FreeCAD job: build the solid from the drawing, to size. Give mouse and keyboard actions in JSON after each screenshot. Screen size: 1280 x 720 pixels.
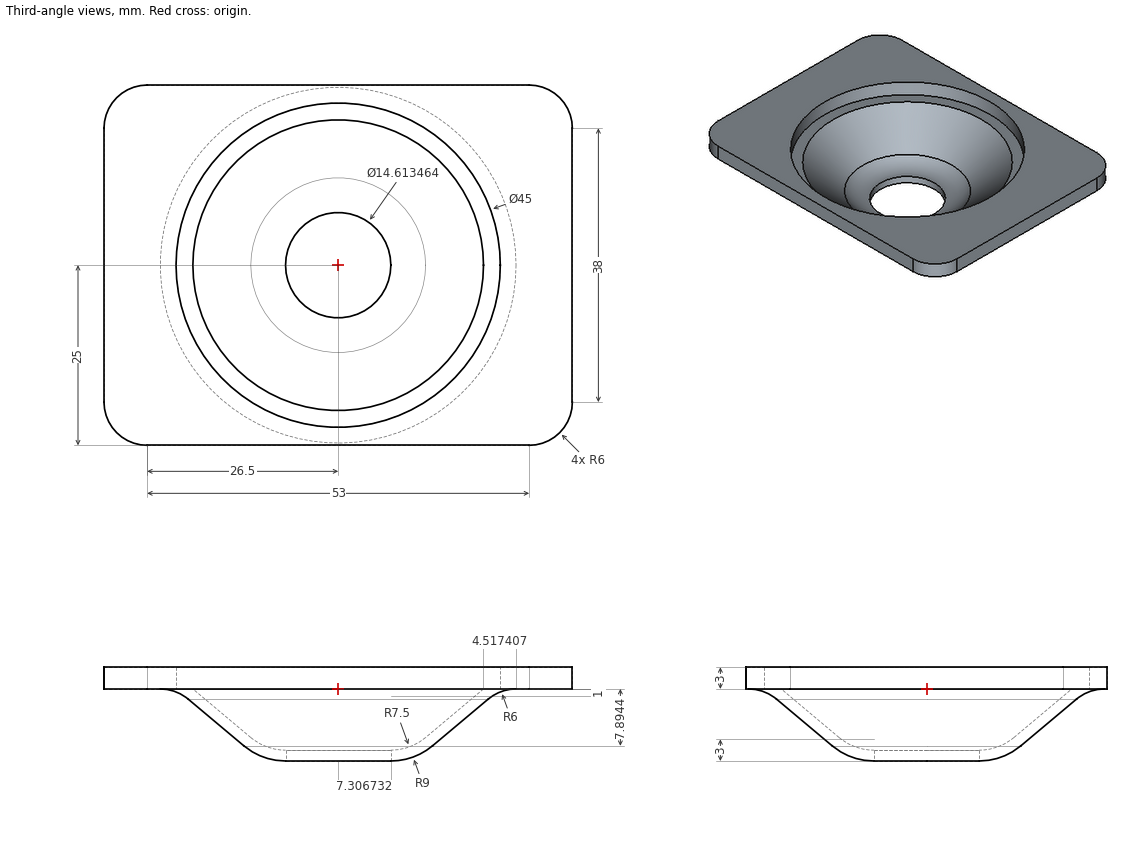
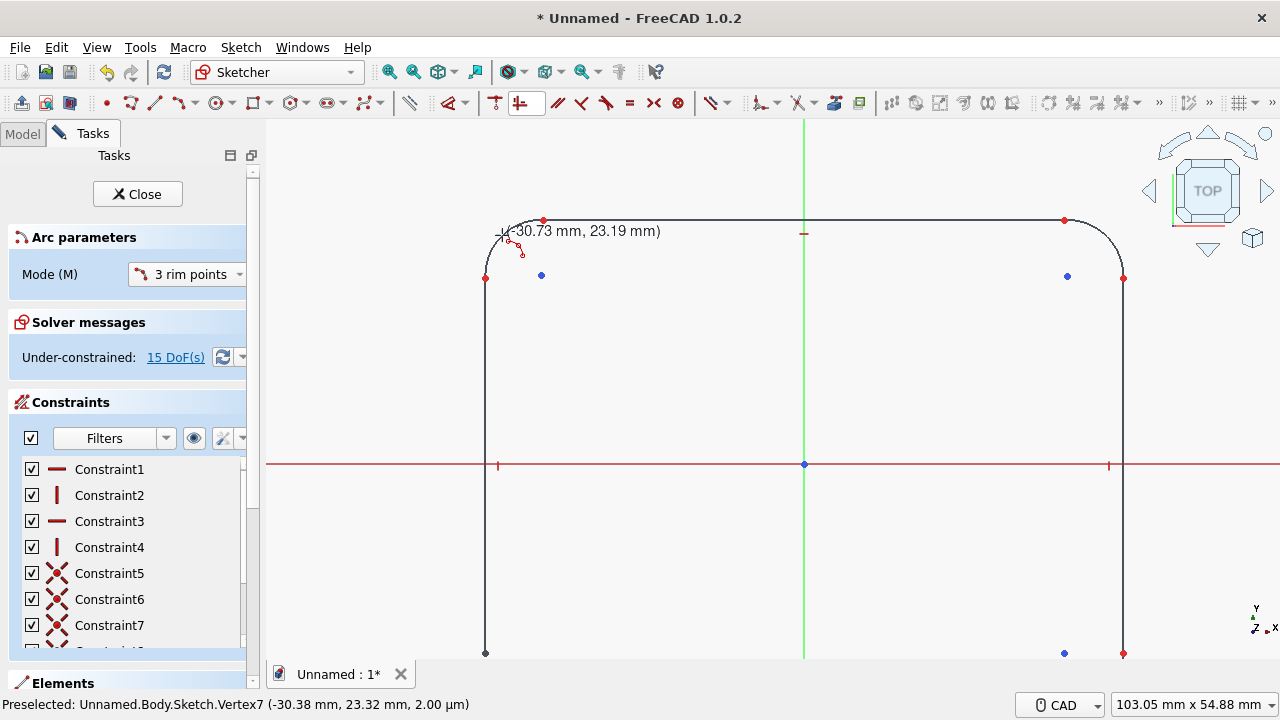
{"action": "scroll", "coordinate": [501, 236], "scroll_direction": "down", "scroll_amount": 2}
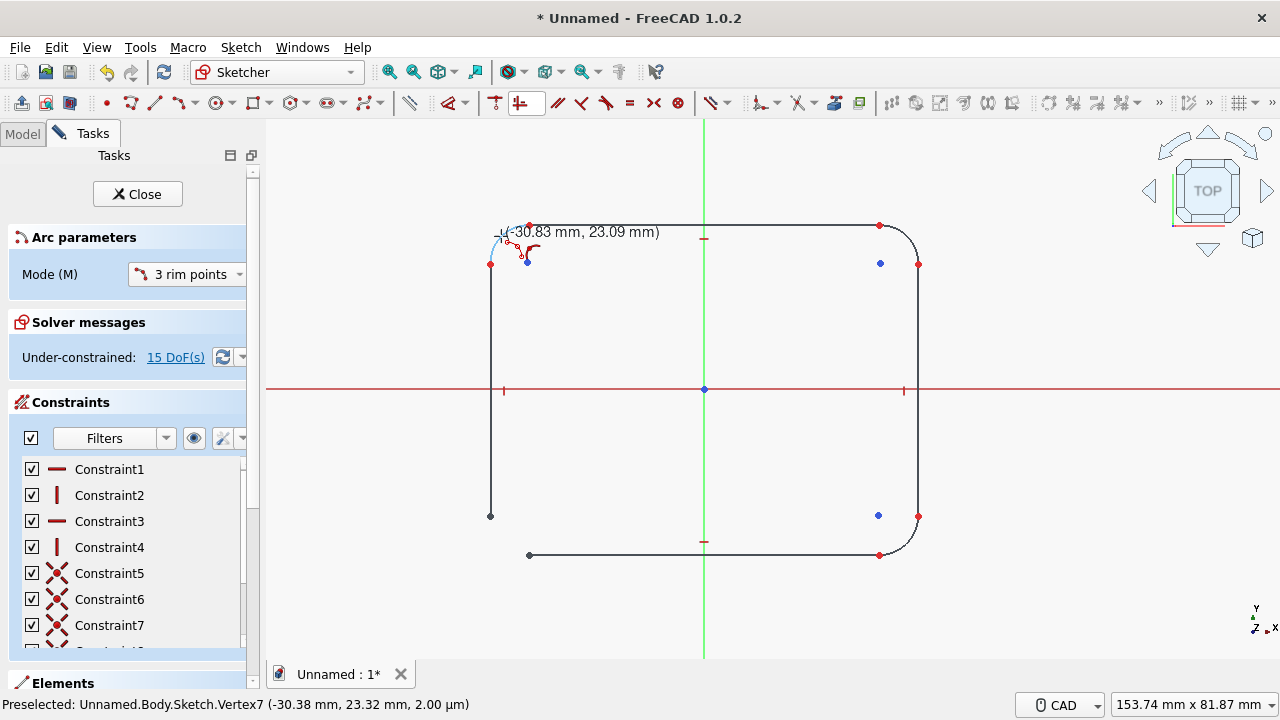
{"action": "left_click", "coordinate": [491, 516]}
{"action": "left_click", "coordinate": [530, 555]}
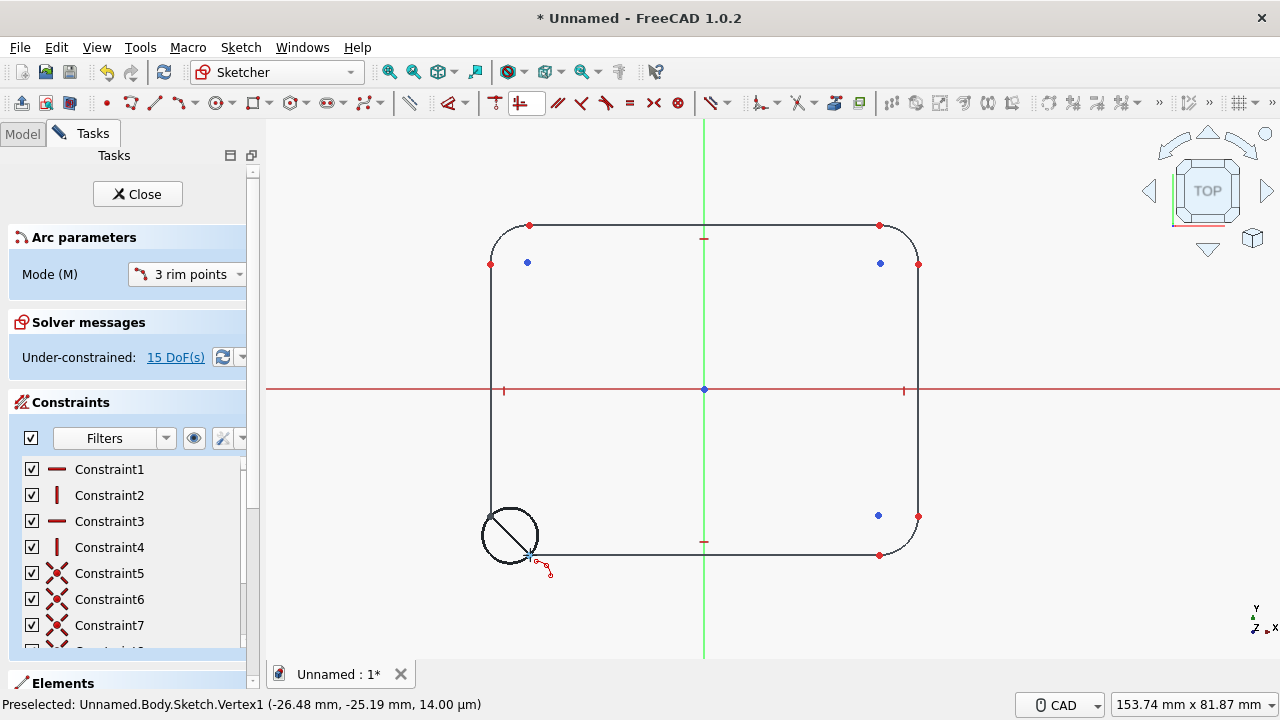
{"action": "scroll", "coordinate": [502, 542], "scroll_direction": "up", "scroll_amount": 2}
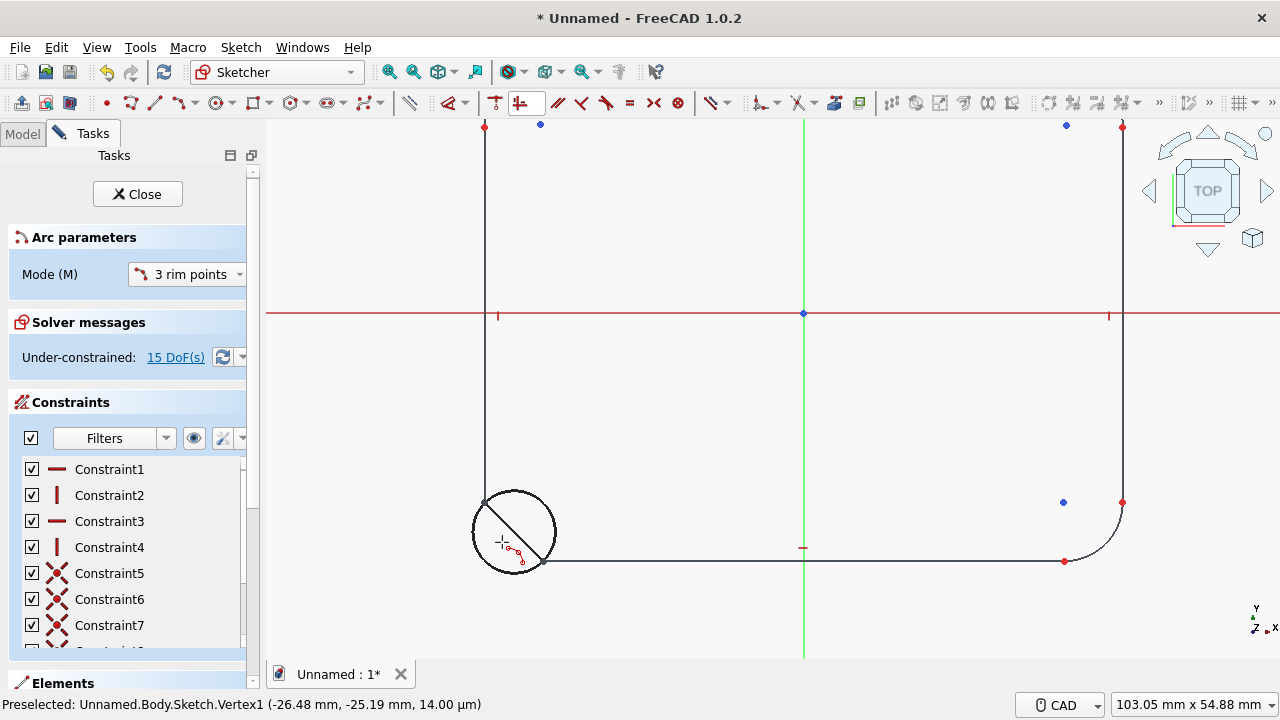
{"action": "left_click", "coordinate": [501, 542]}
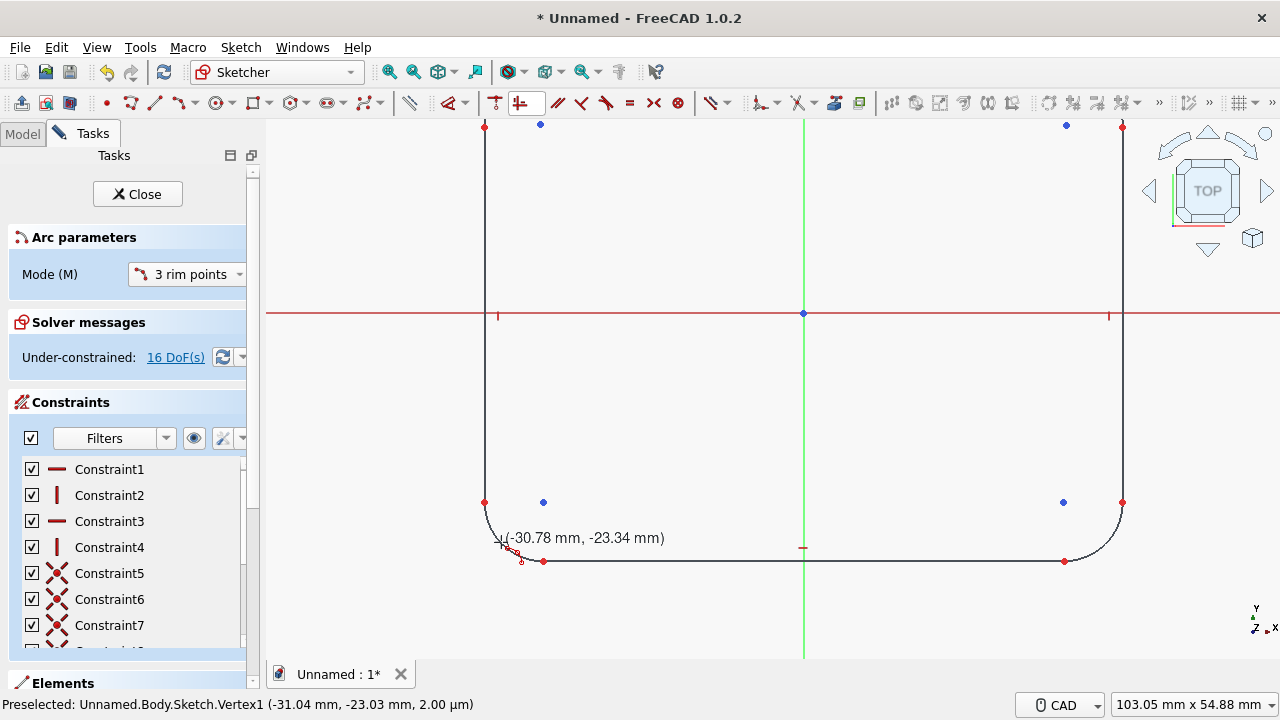
{"action": "key", "text": "g c"}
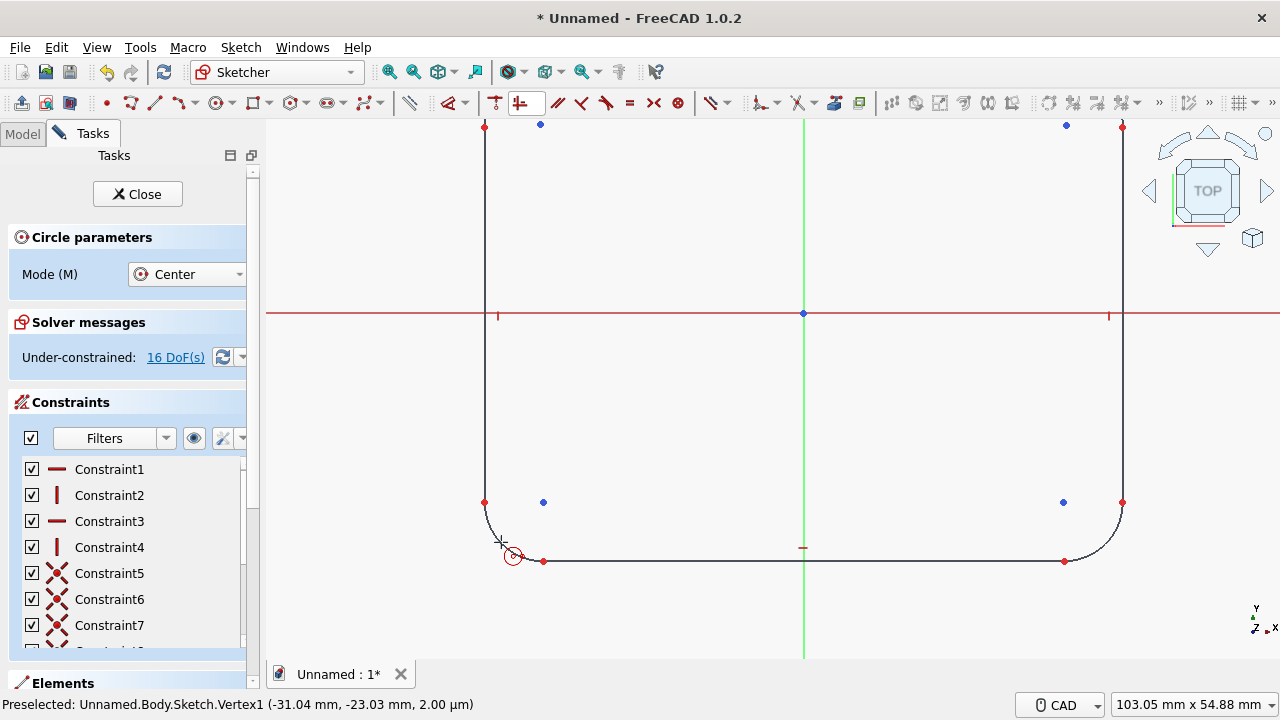
{"action": "left_click", "coordinate": [804, 313]}
{"action": "mouse_move", "coordinate": [960, 157]}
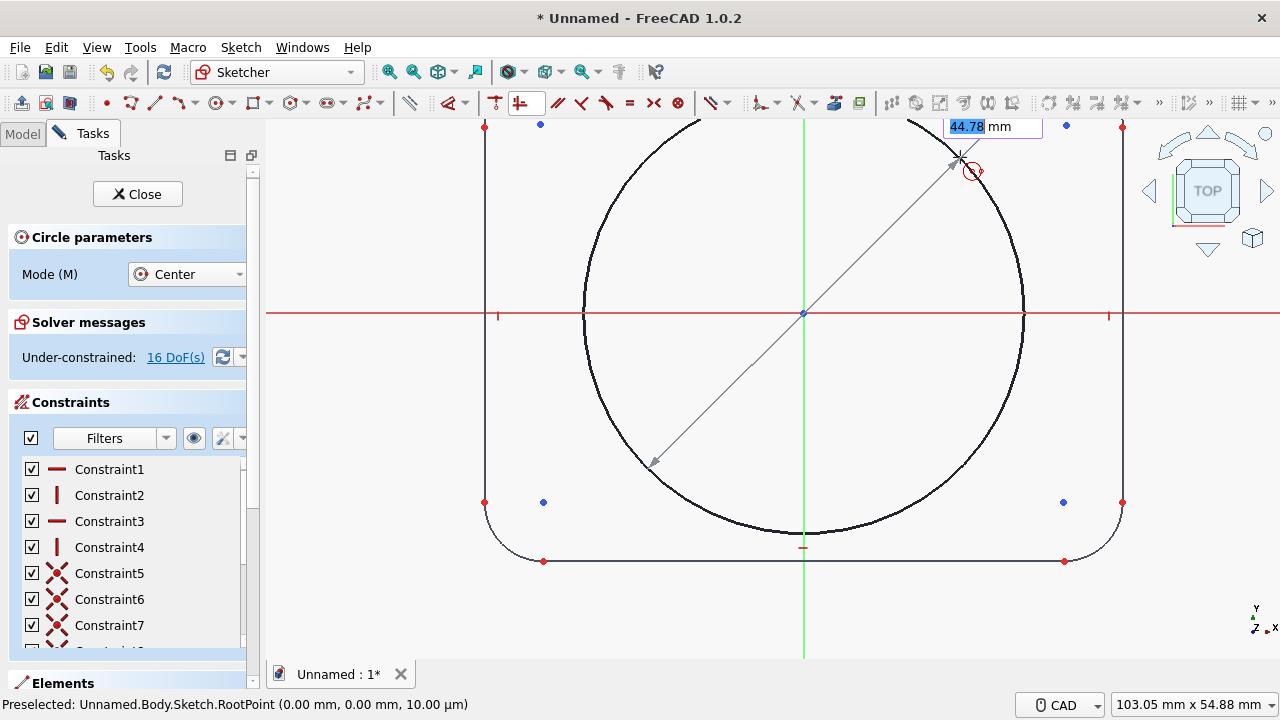
{"action": "type", "text": "45"}
{"action": "key", "text": "Return"}
{"action": "key", "text": "Escape"}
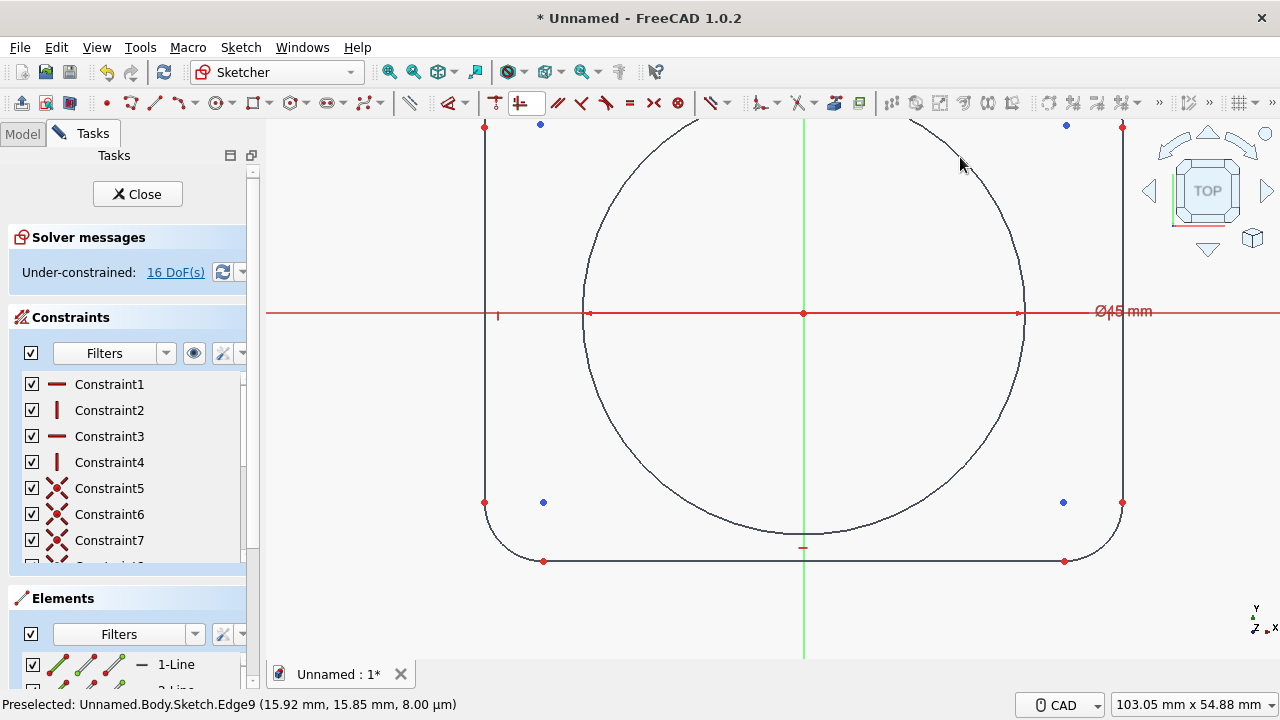
{"action": "left_click", "coordinate": [700, 561]}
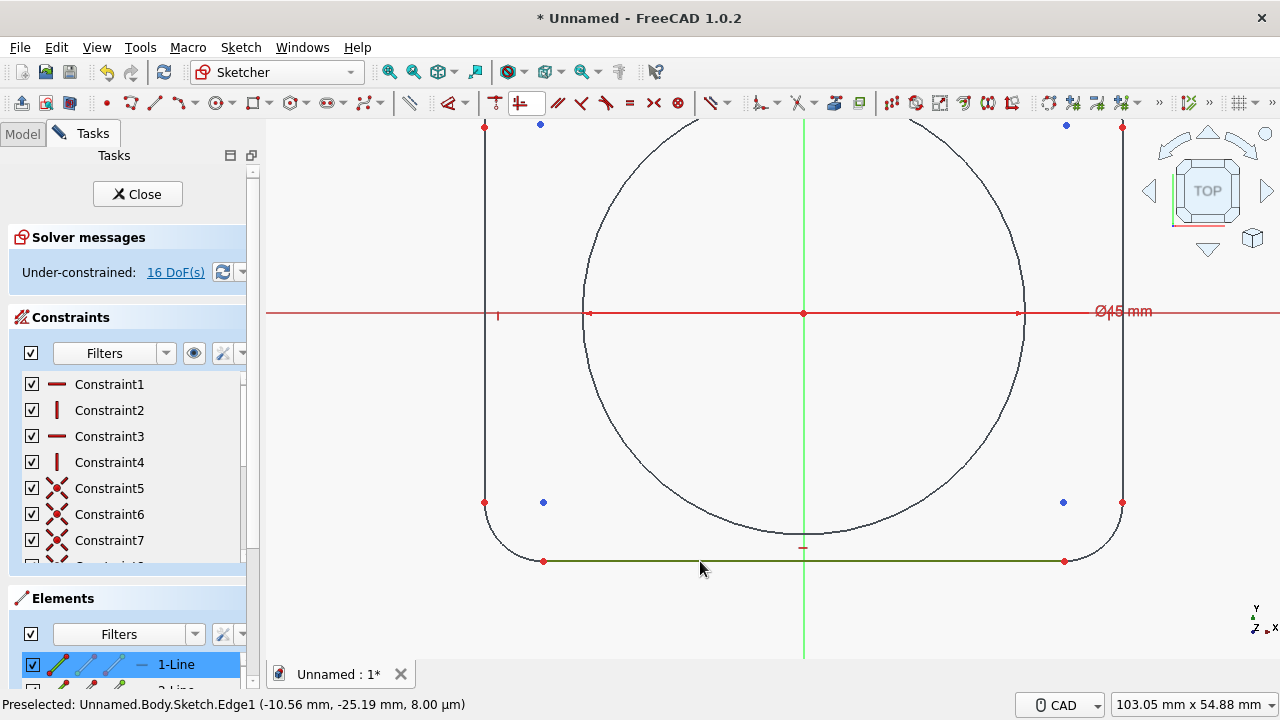
{"action": "left_click", "coordinate": [1091, 555]}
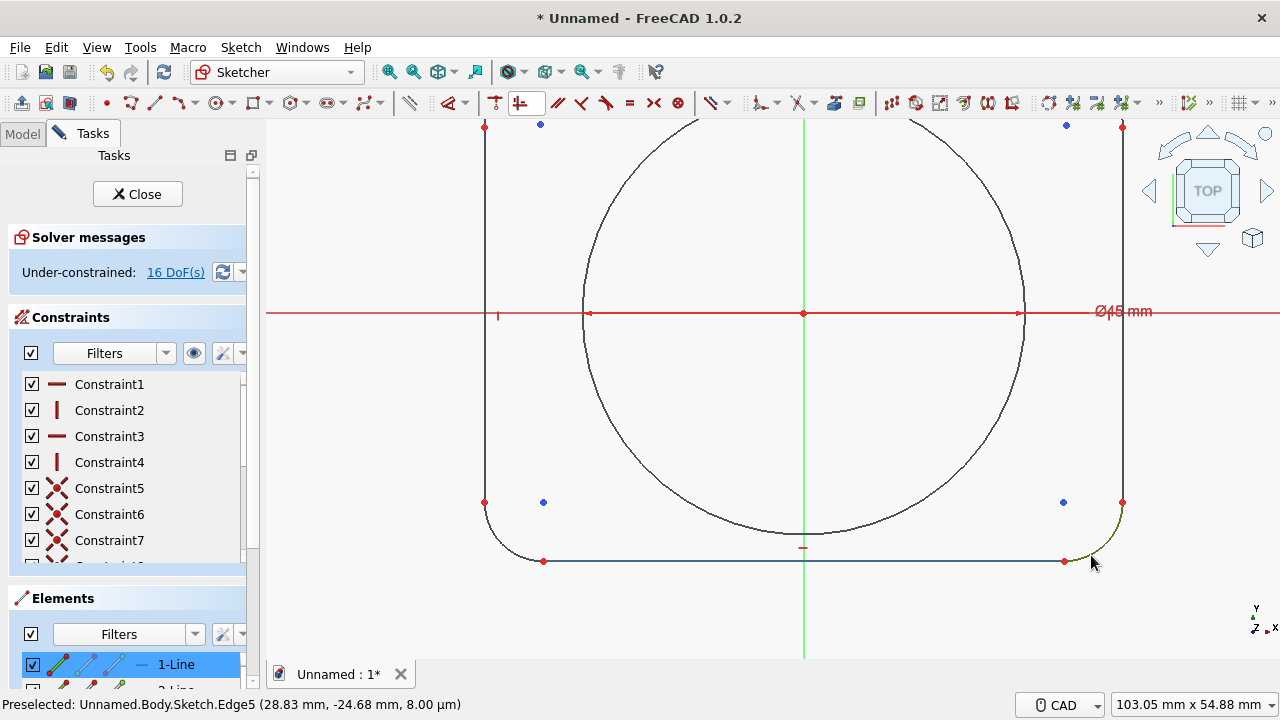
{"action": "key", "text": "t"}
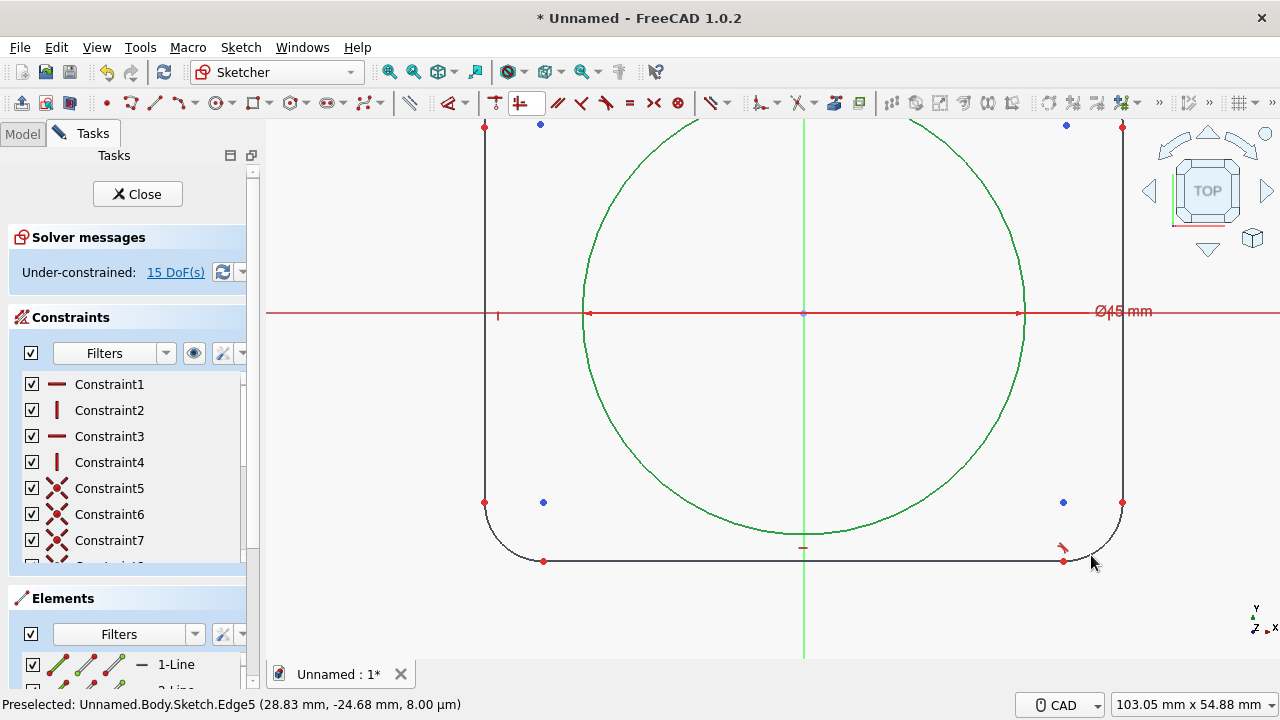
{"action": "left_click", "coordinate": [699, 561]}